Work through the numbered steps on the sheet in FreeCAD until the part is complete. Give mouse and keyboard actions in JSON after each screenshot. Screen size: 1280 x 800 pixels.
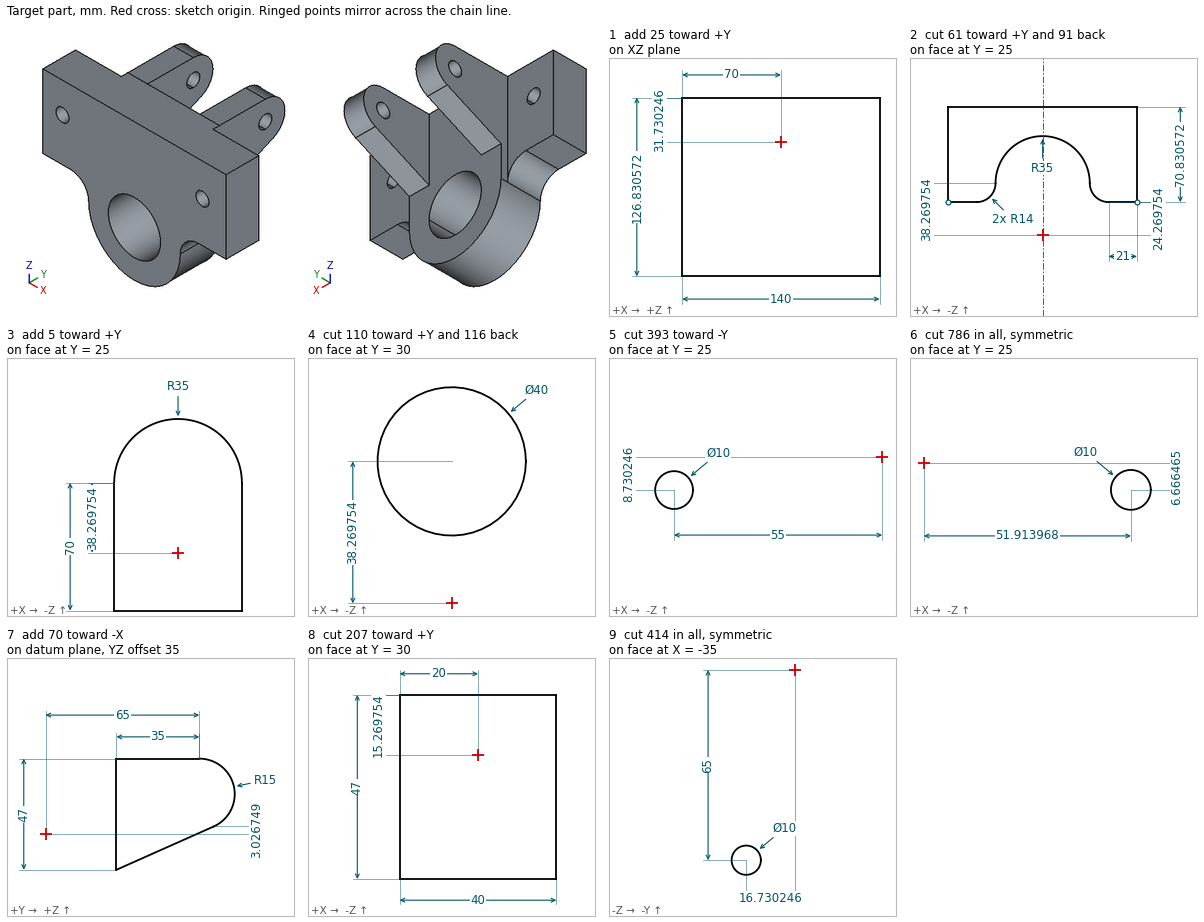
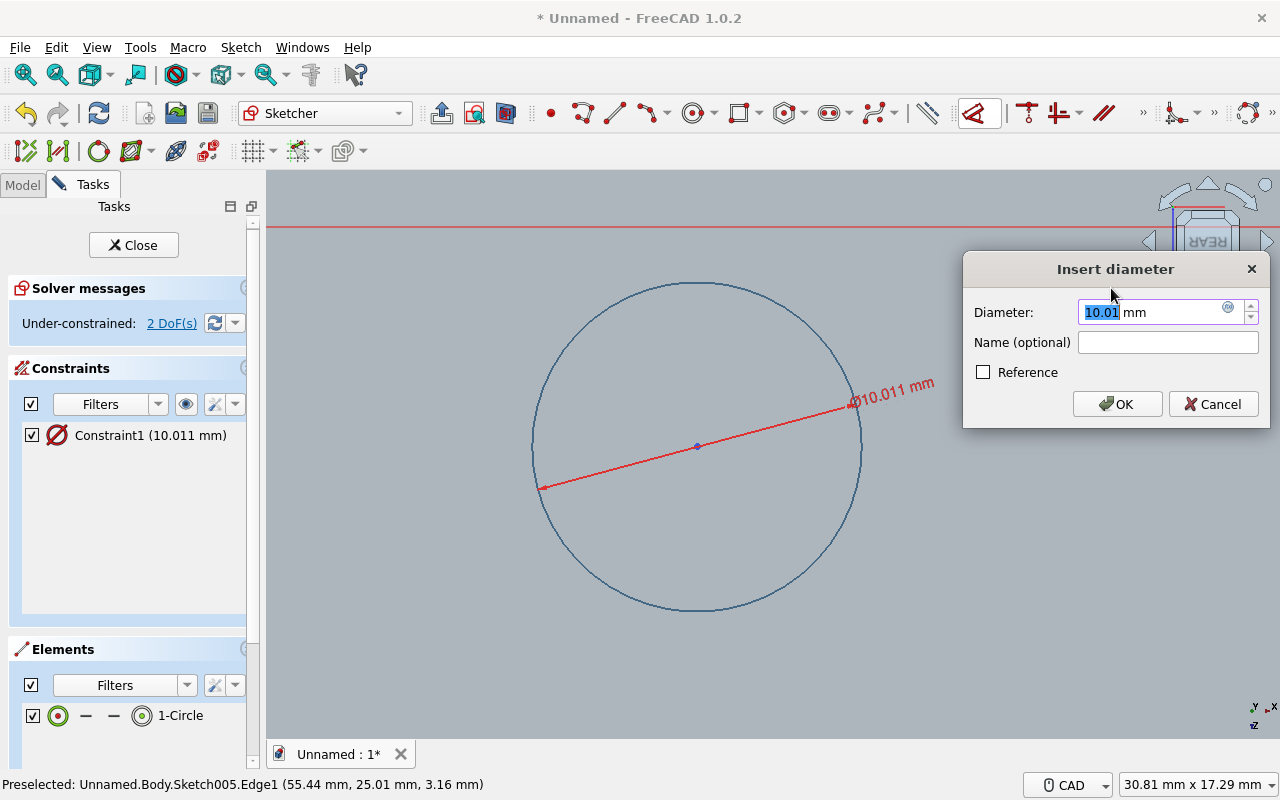
{"action": "type", "text": "10"}
{"action": "key", "text": "Return"}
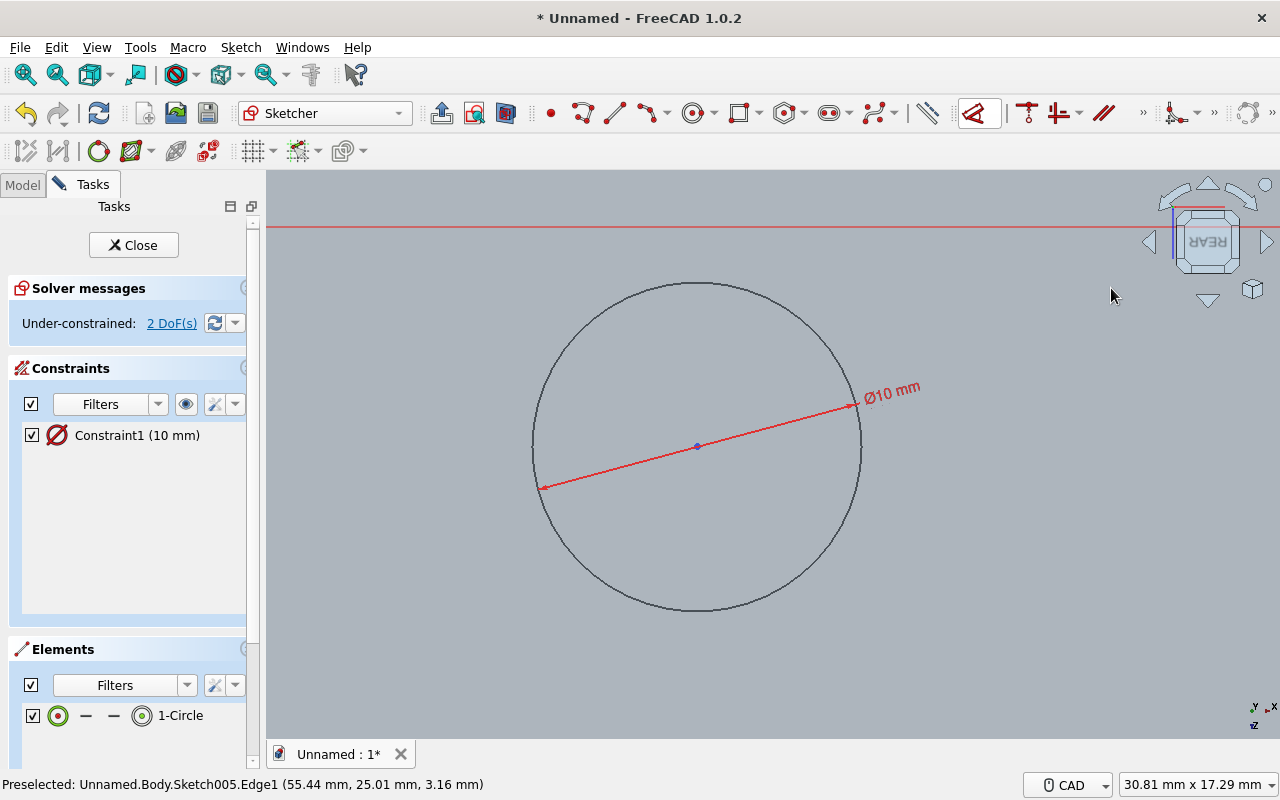
{"action": "left_click", "coordinate": [697, 447]}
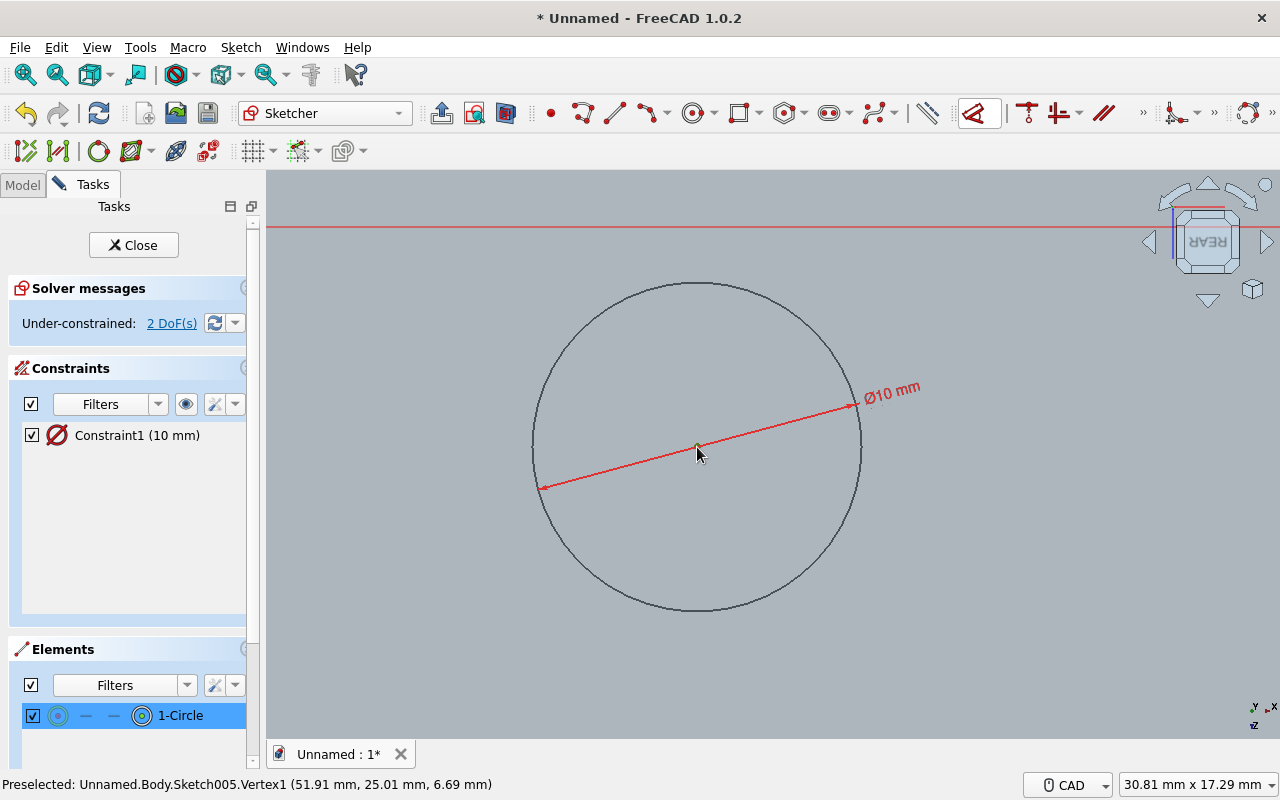
{"action": "key", "text": "i"}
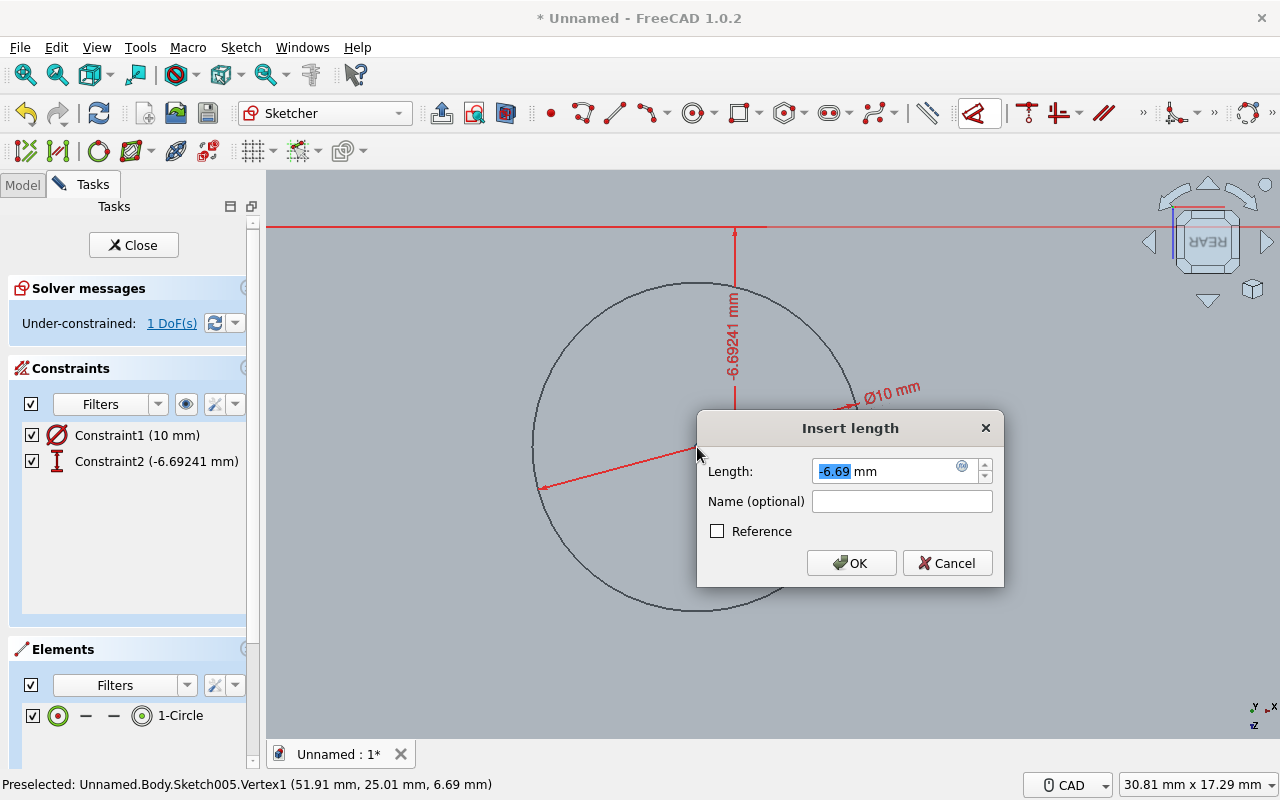
{"action": "type", "text": "-6.666465"}
{"action": "key", "text": "Return"}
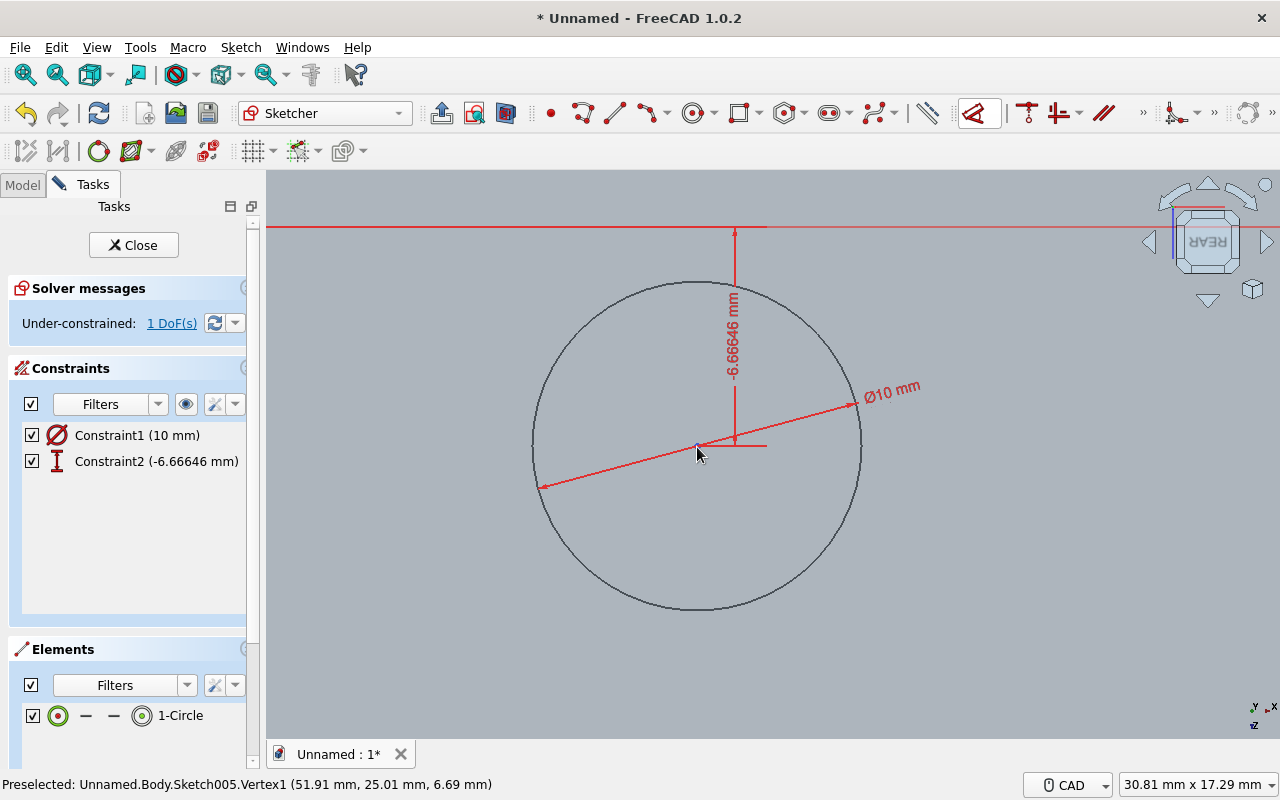
{"action": "left_click", "coordinate": [697, 446]}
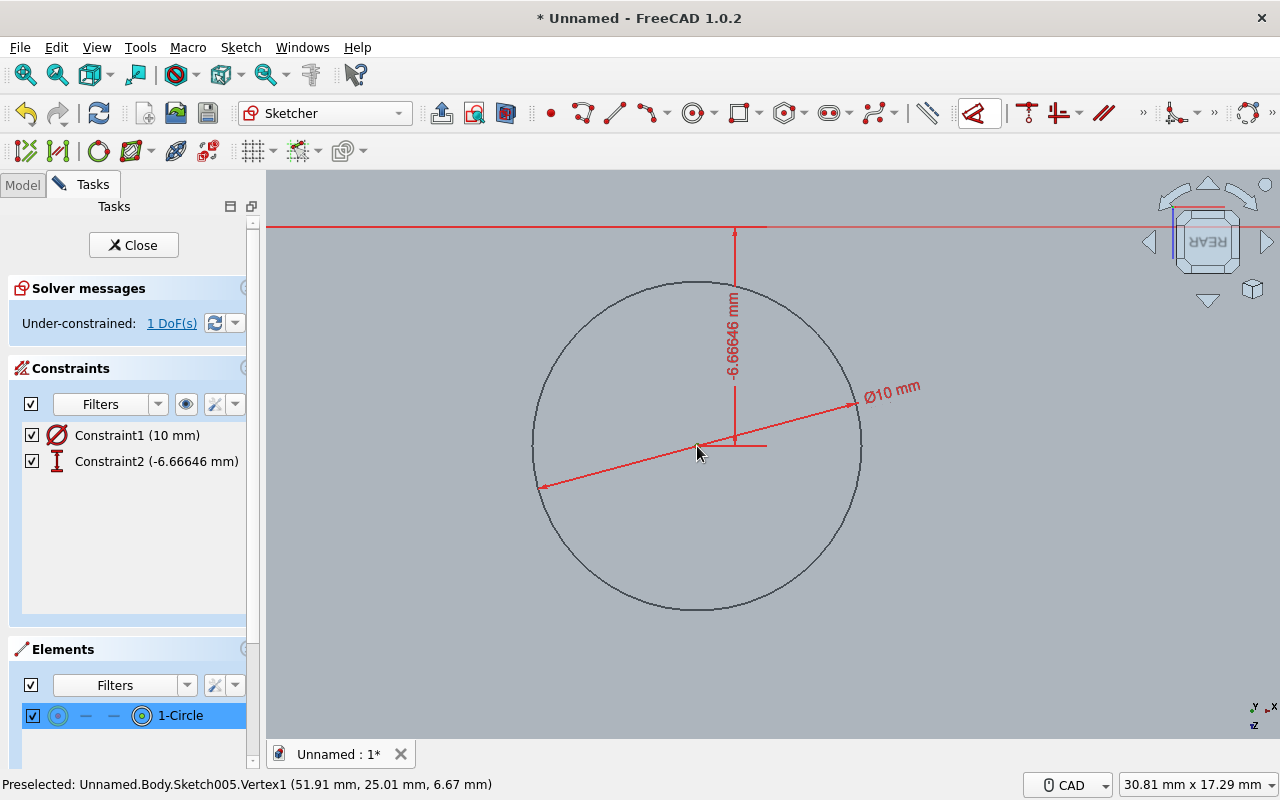
{"action": "key", "text": "l"}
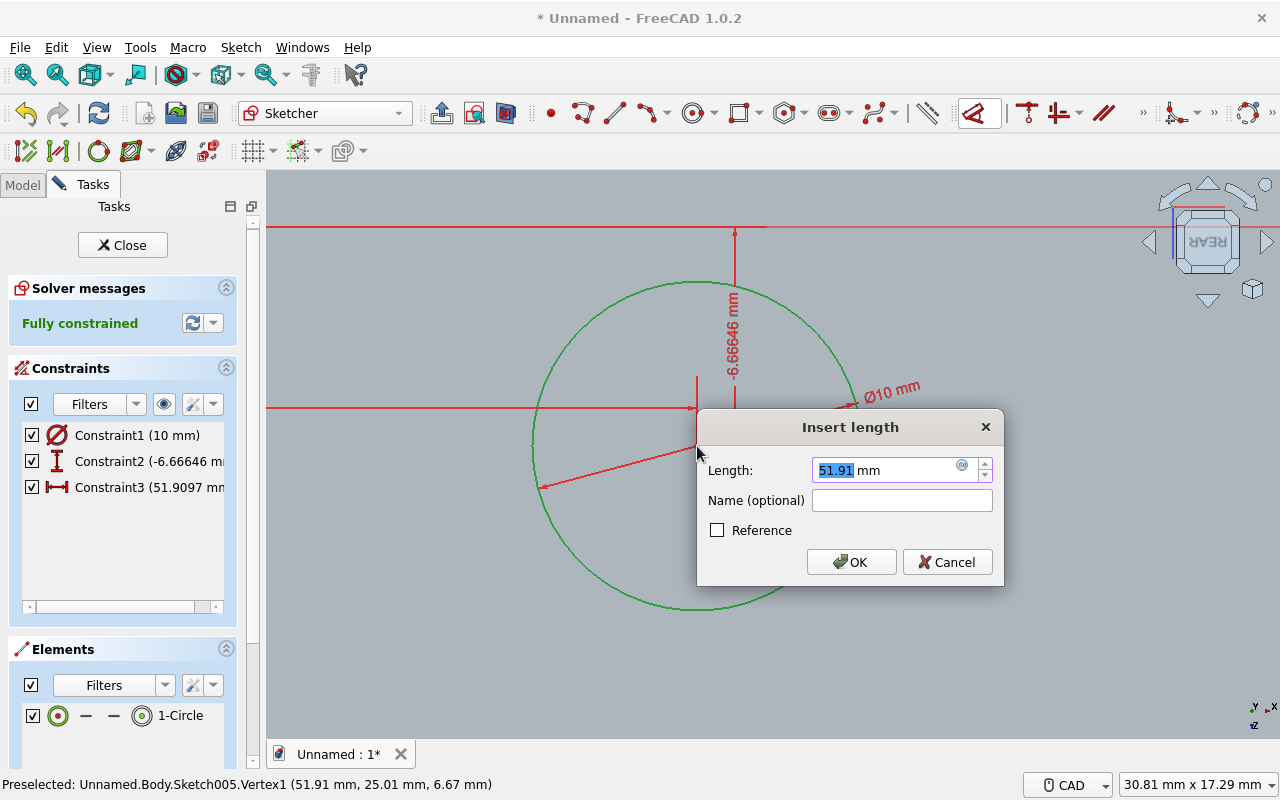
{"action": "type", "text": "51.913968"}
{"action": "key", "text": "Return"}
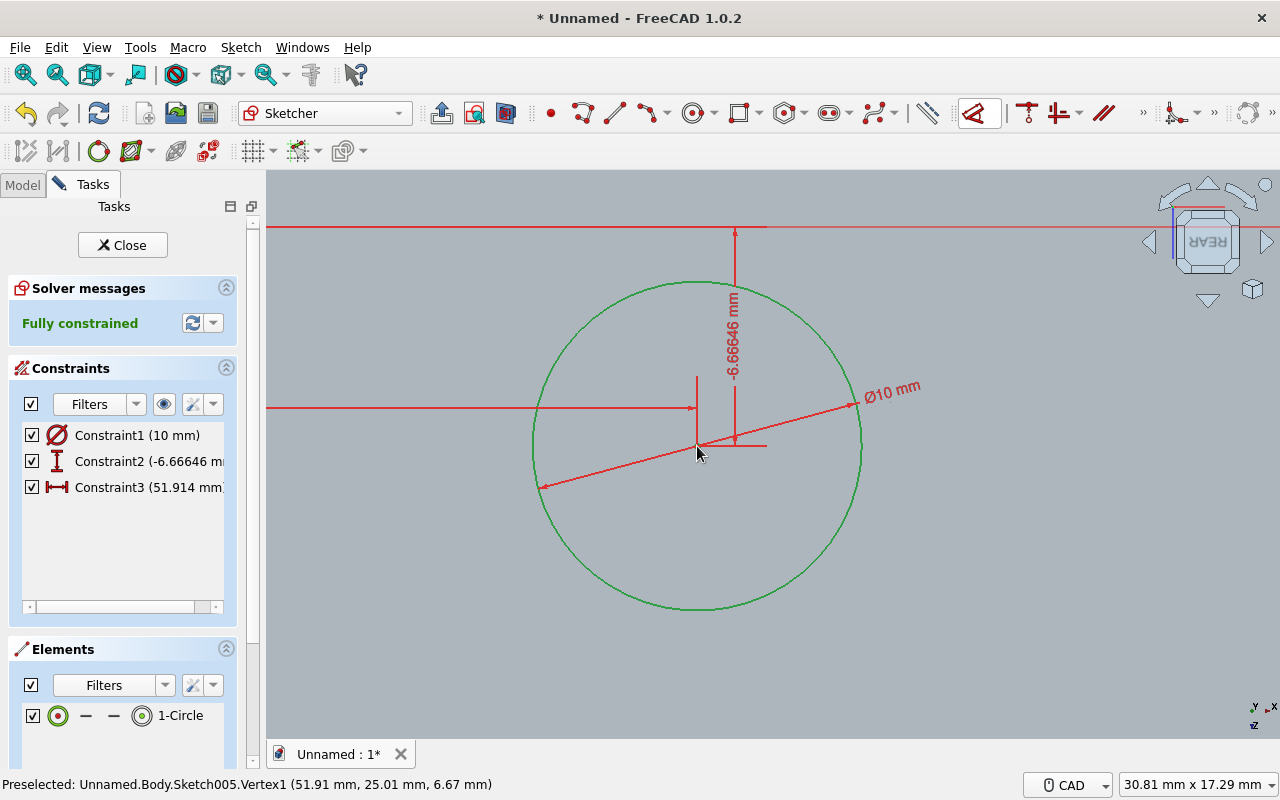
{"action": "left_click", "coordinate": [123, 245]}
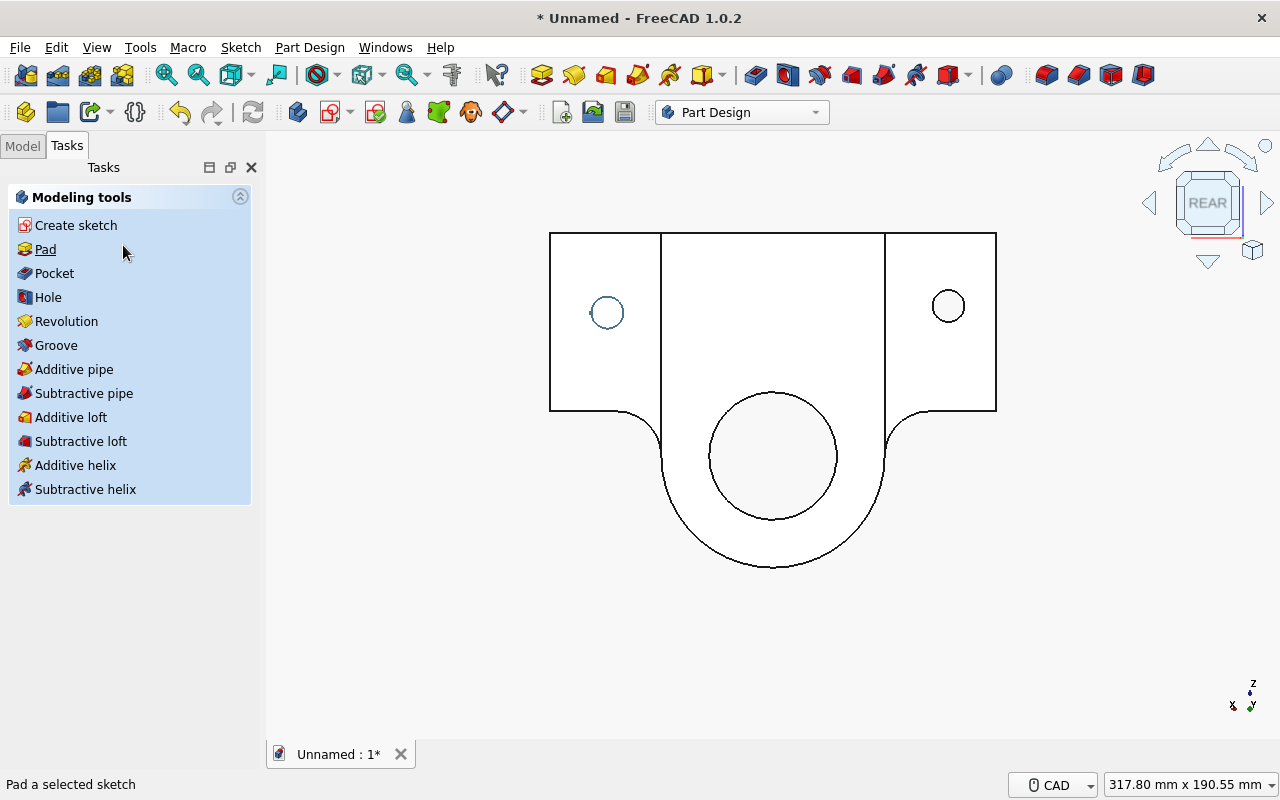
{"action": "left_click", "coordinate": [756, 76]}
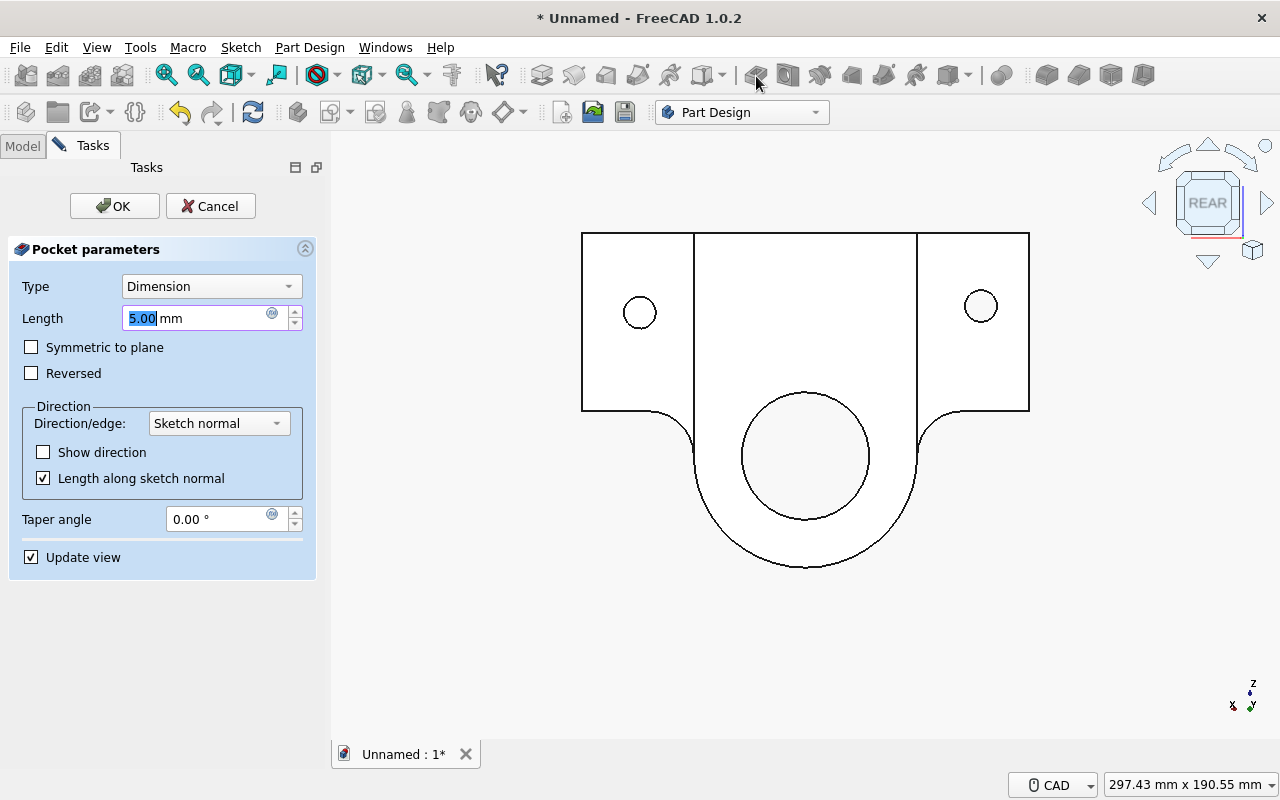
{"action": "type", "text": "786"}
{"action": "key", "text": "Tab"}